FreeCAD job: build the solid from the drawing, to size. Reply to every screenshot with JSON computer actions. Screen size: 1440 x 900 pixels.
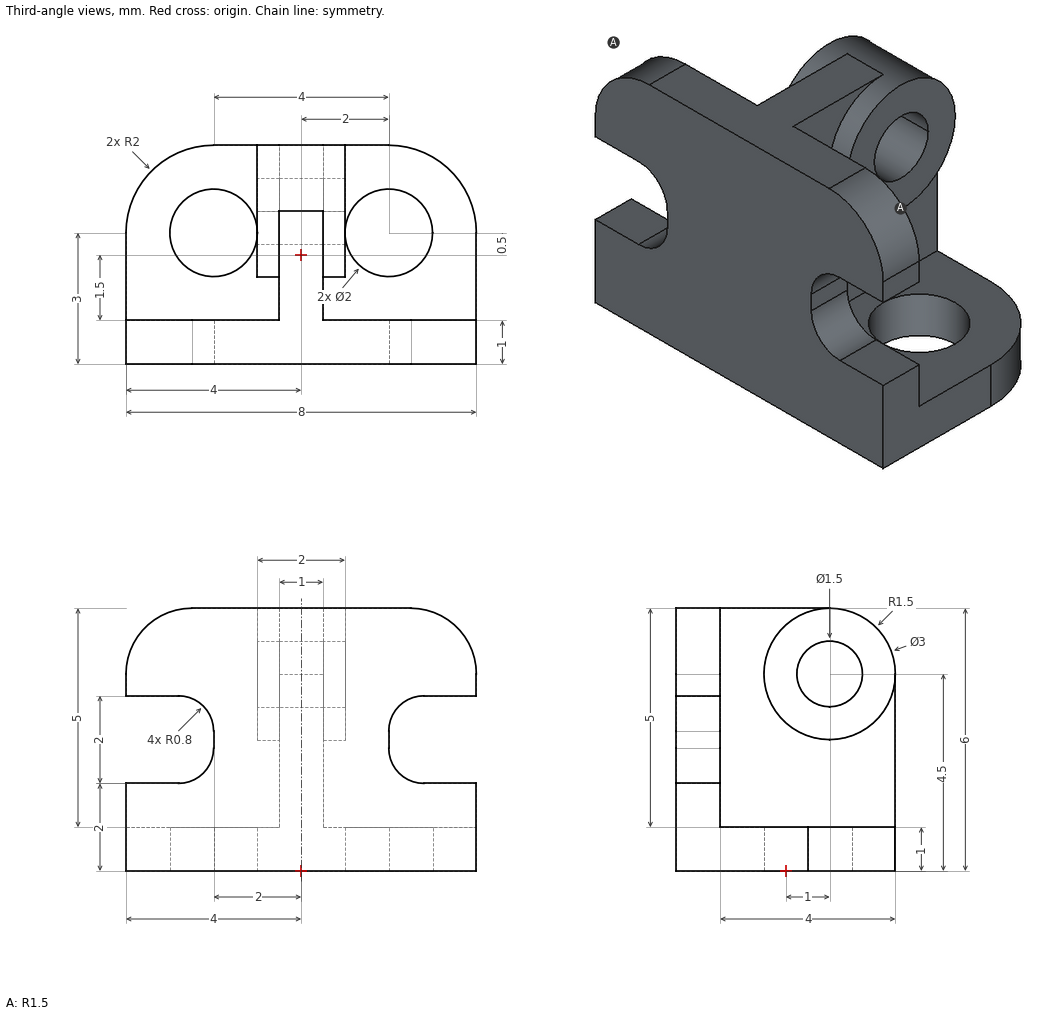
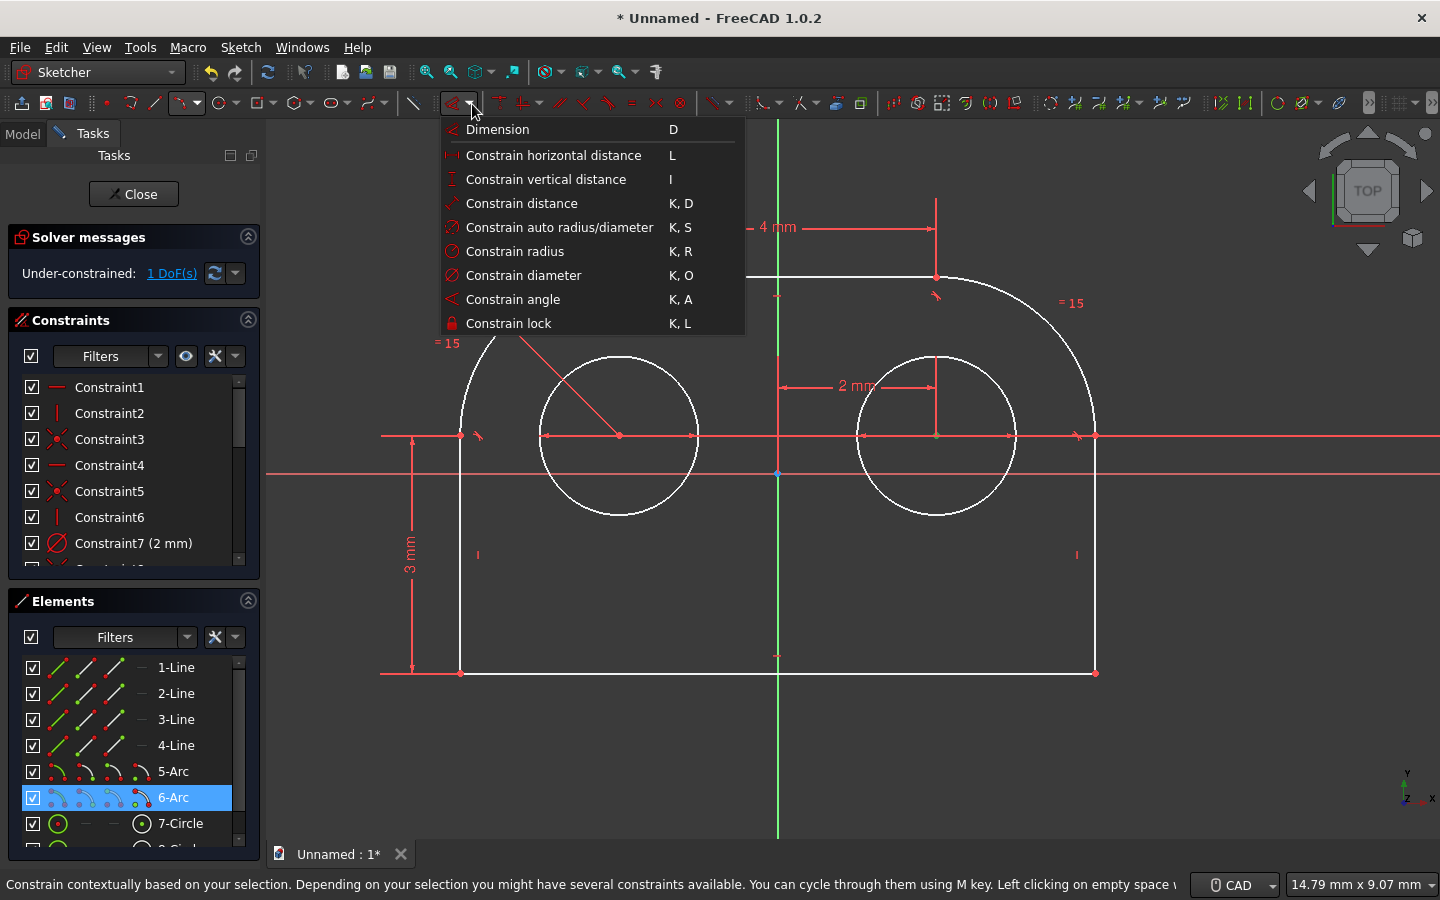
{"action": "left_click", "coordinate": [593, 179]}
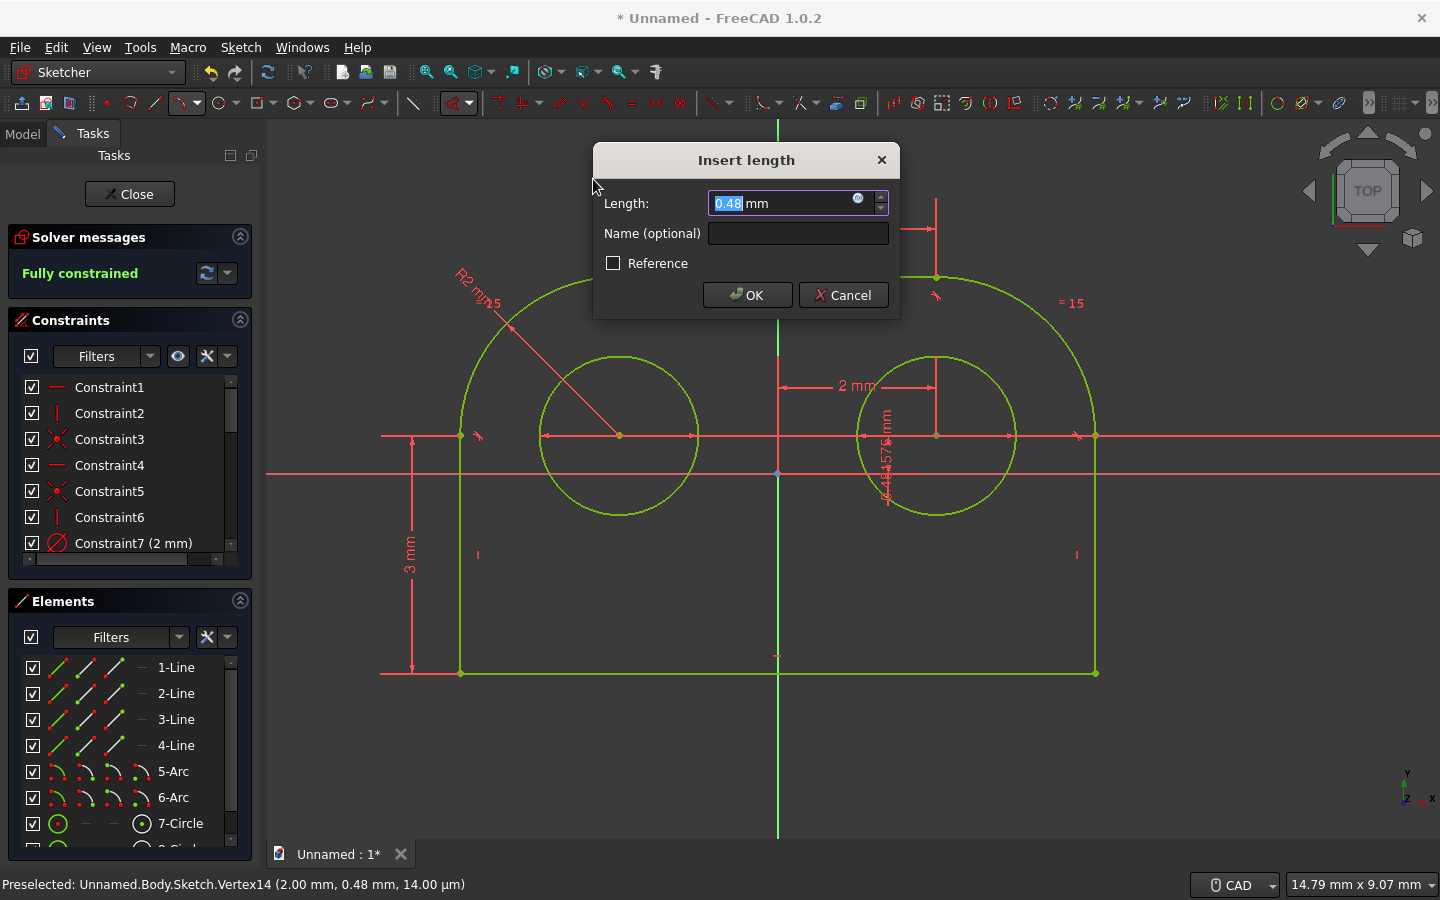
{"action": "type", "text": "0.5"}
{"action": "key", "text": "Return"}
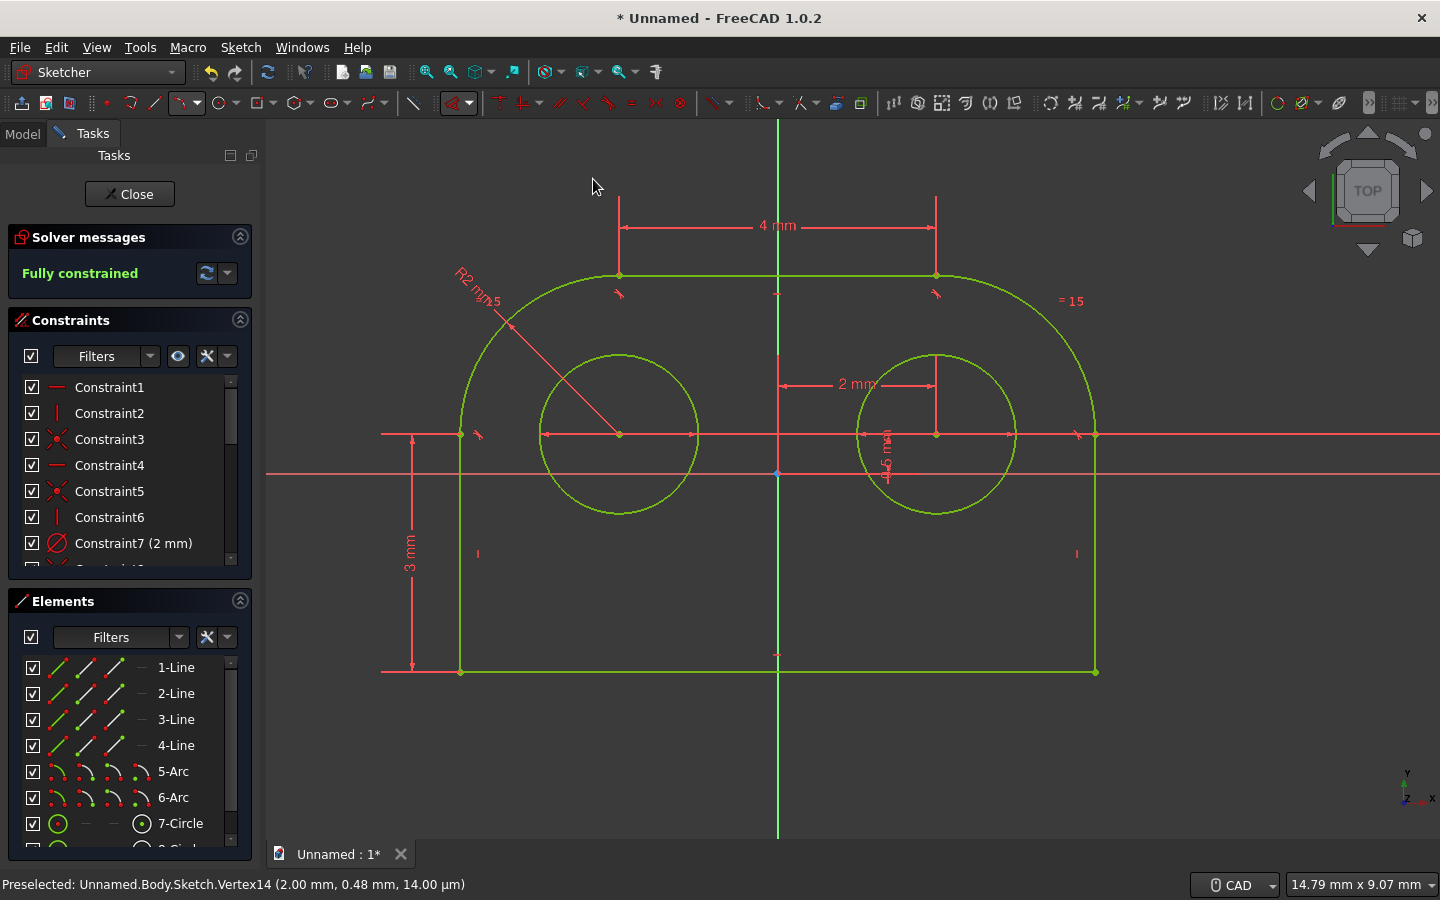
{"action": "left_click", "coordinate": [130, 194]}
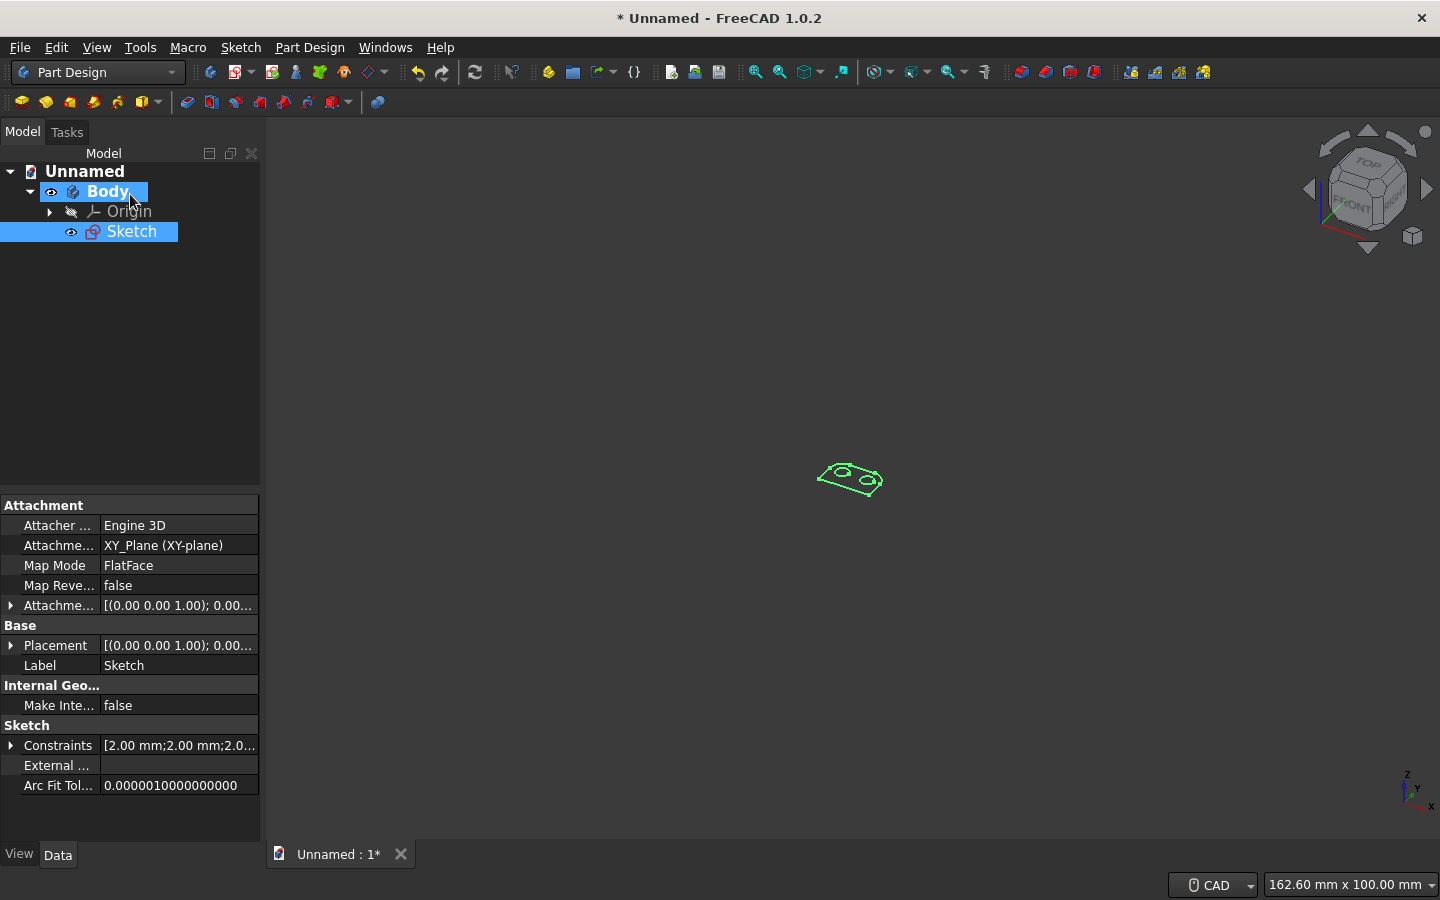
{"action": "left_click", "coordinate": [22, 102]}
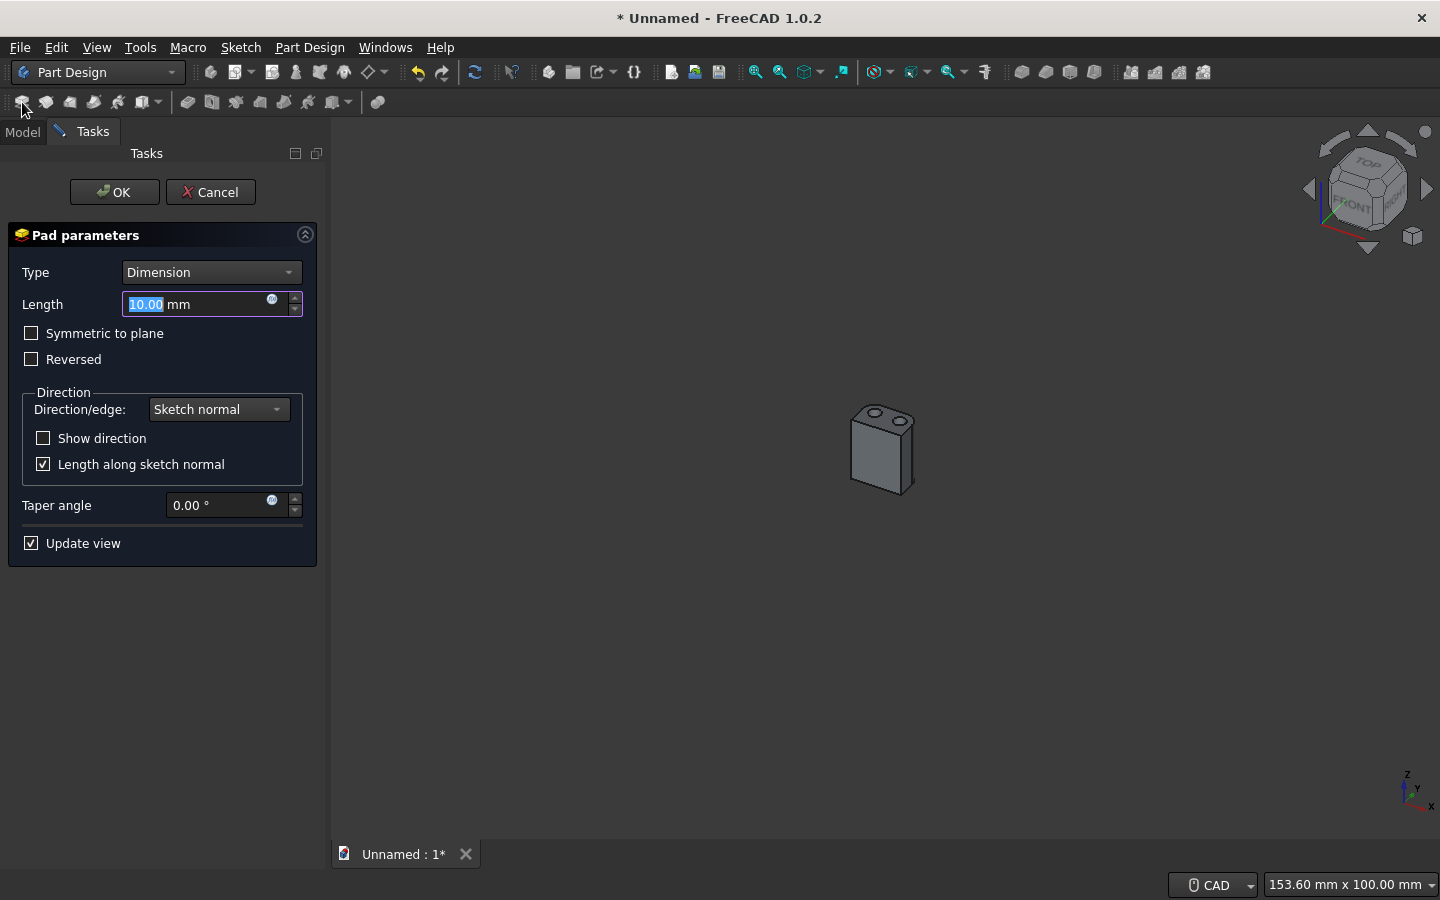
{"action": "type", "text": "1"}
{"action": "key", "text": "Tab"}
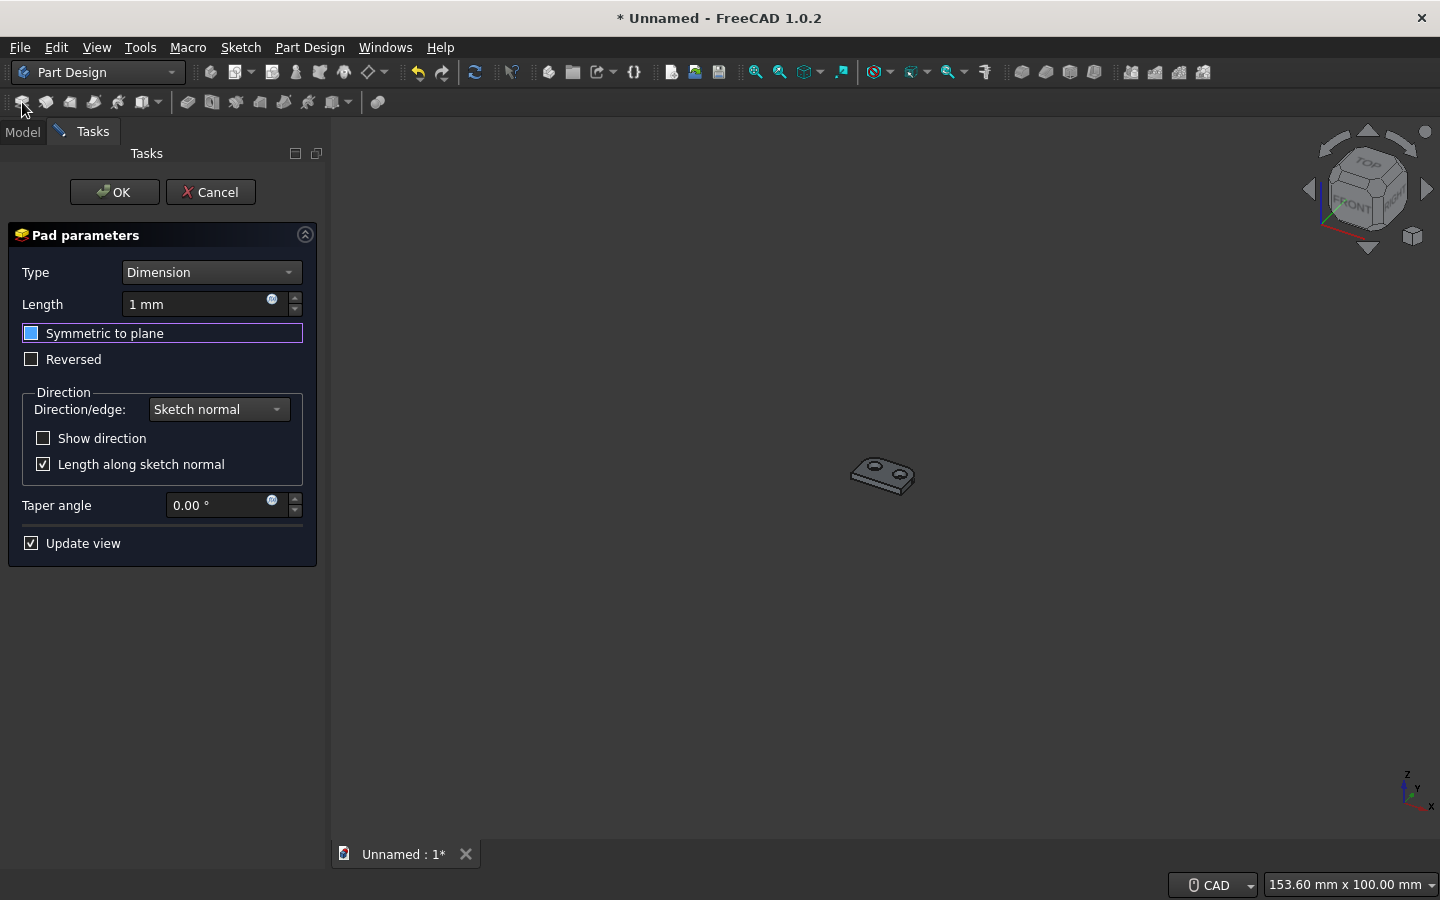
{"action": "left_click", "coordinate": [115, 192]}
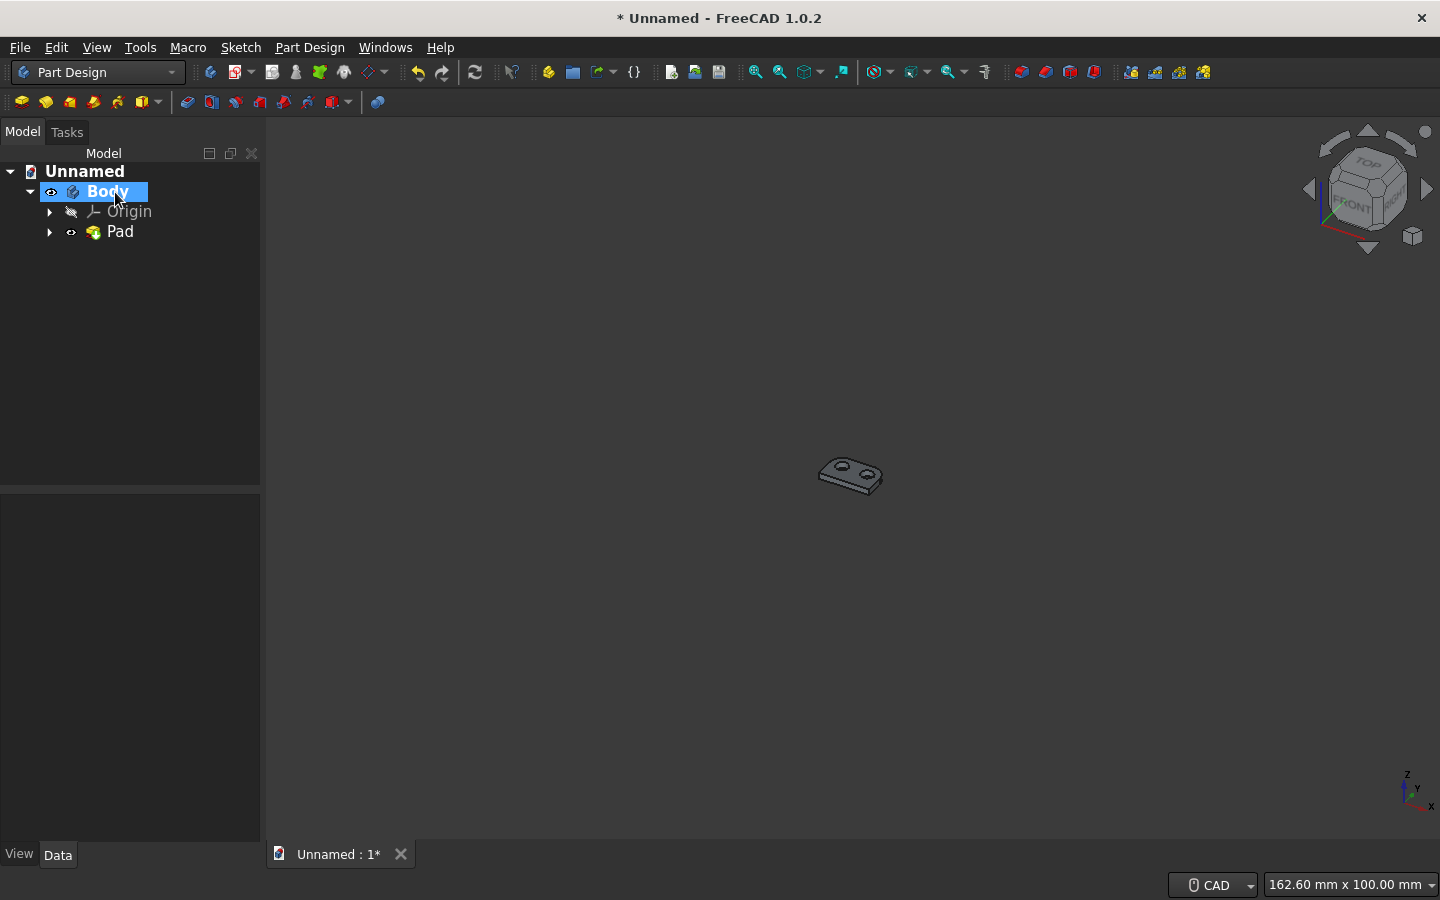
{"action": "left_click", "coordinate": [756, 72]}